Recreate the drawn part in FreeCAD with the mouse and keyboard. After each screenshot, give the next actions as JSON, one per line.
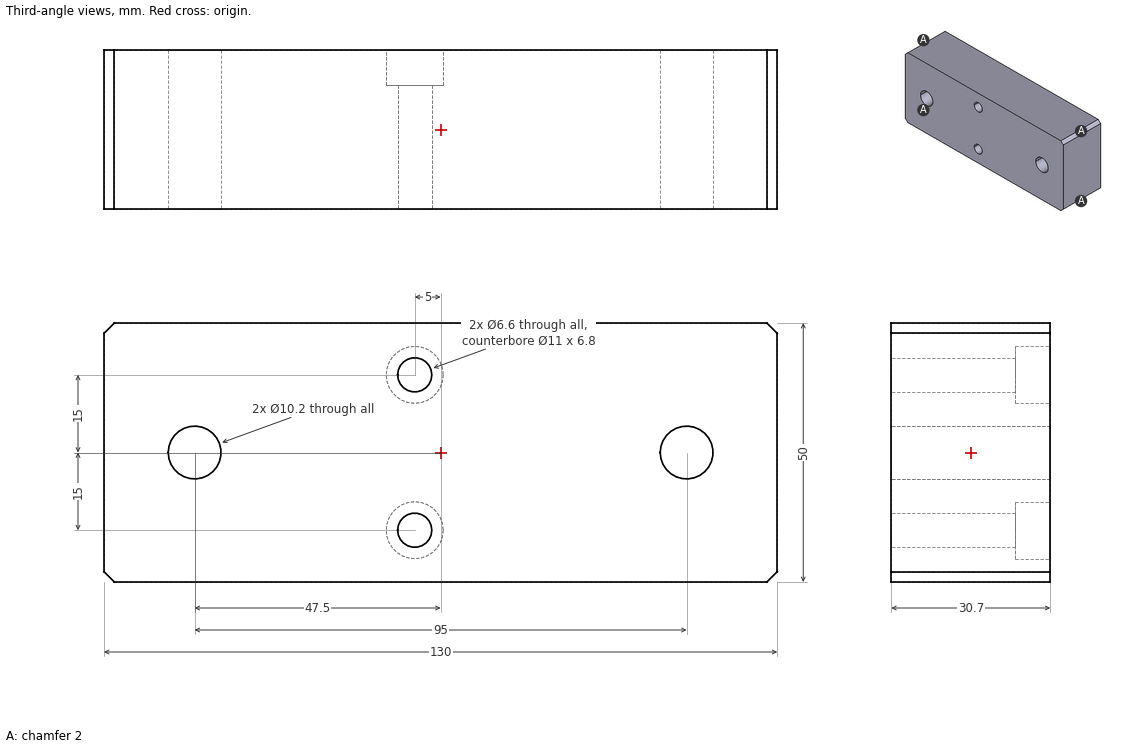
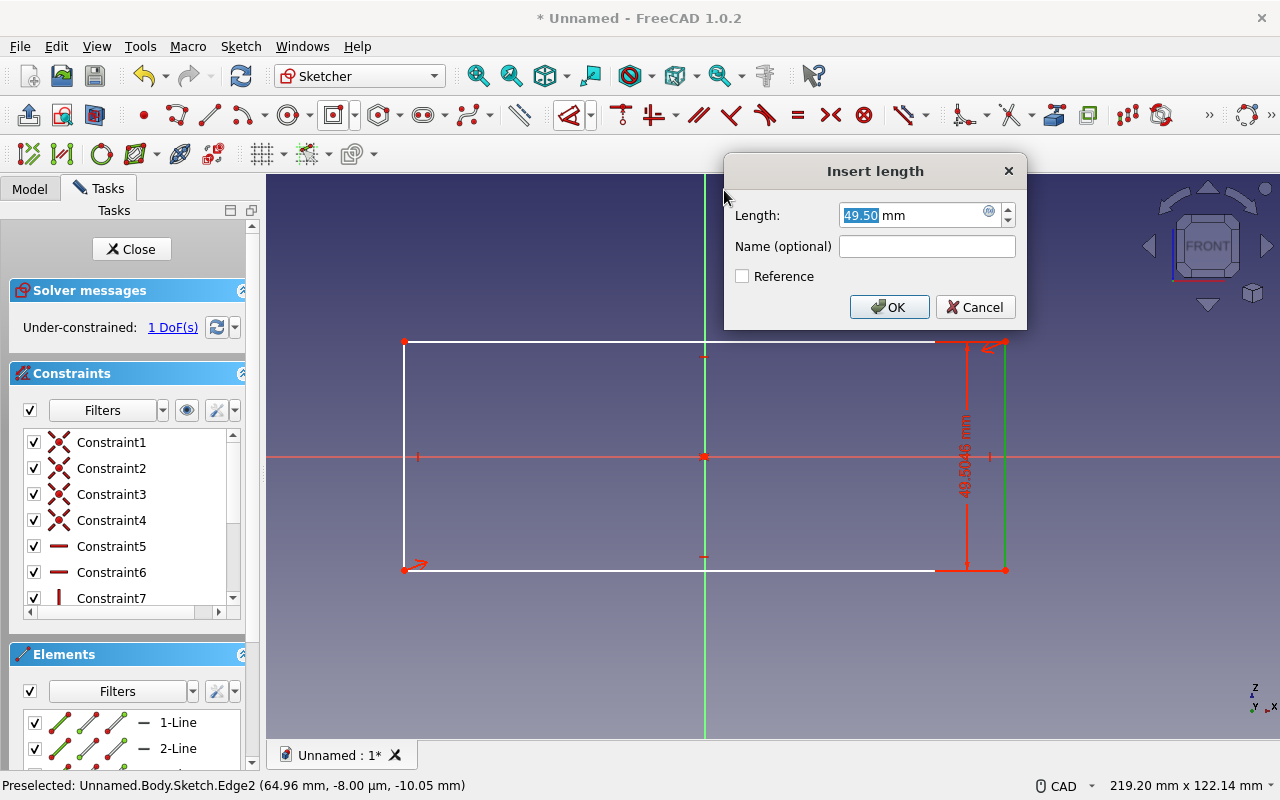
{"action": "type", "text": "50"}
{"action": "key", "text": "Return"}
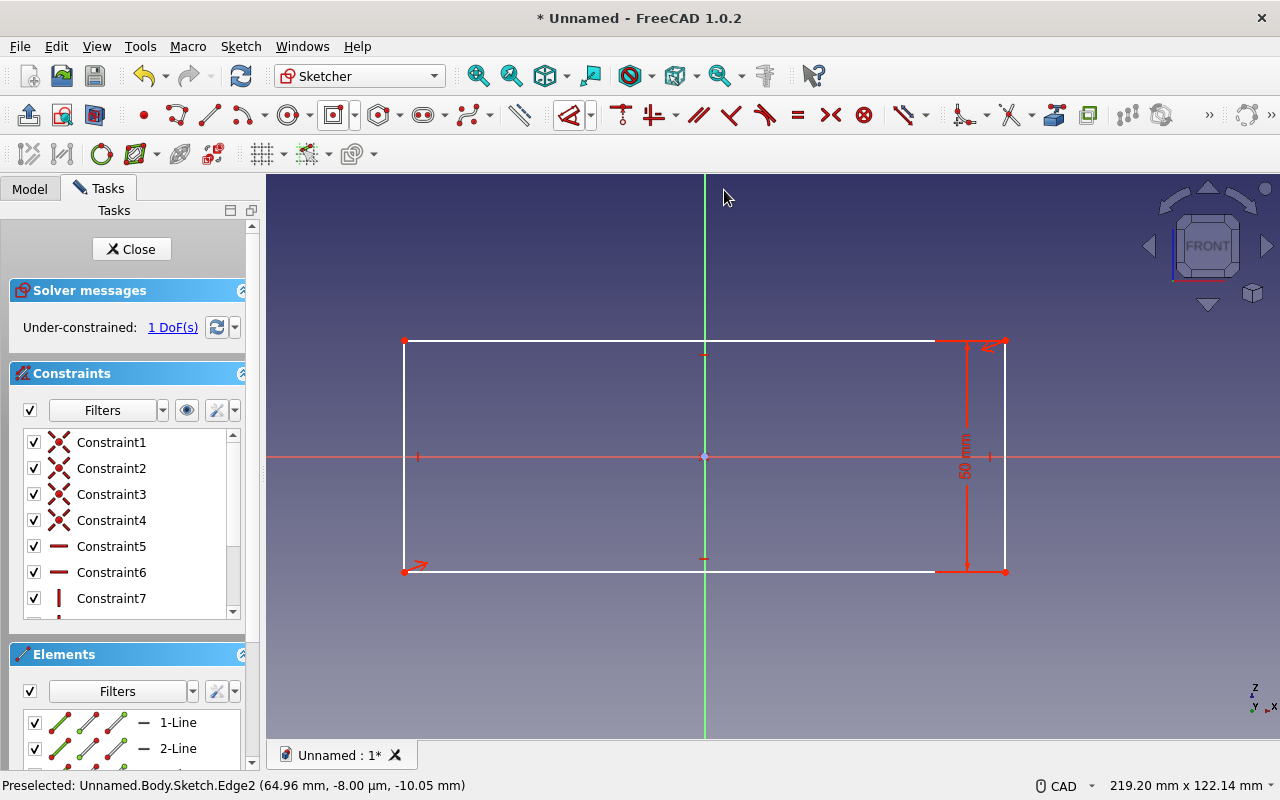
{"action": "left_click", "coordinate": [584, 572]}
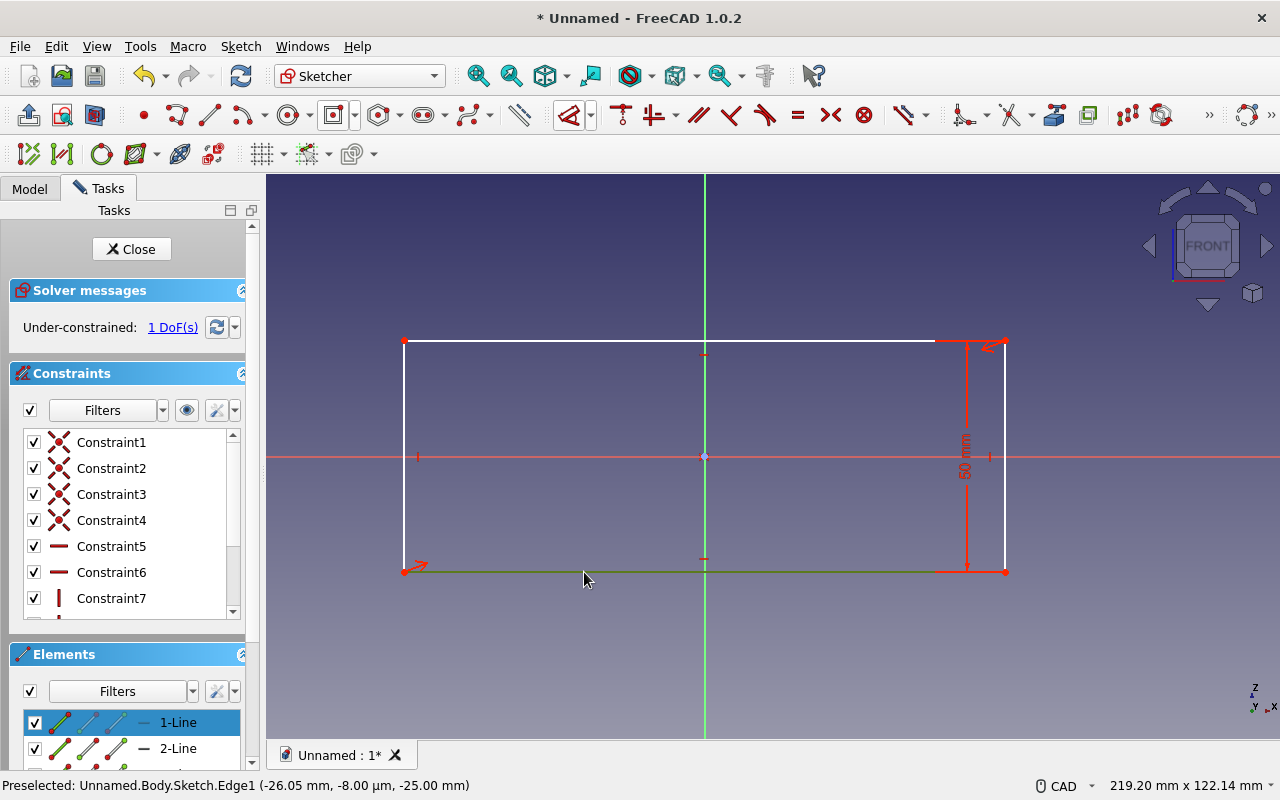
{"action": "key", "text": "l"}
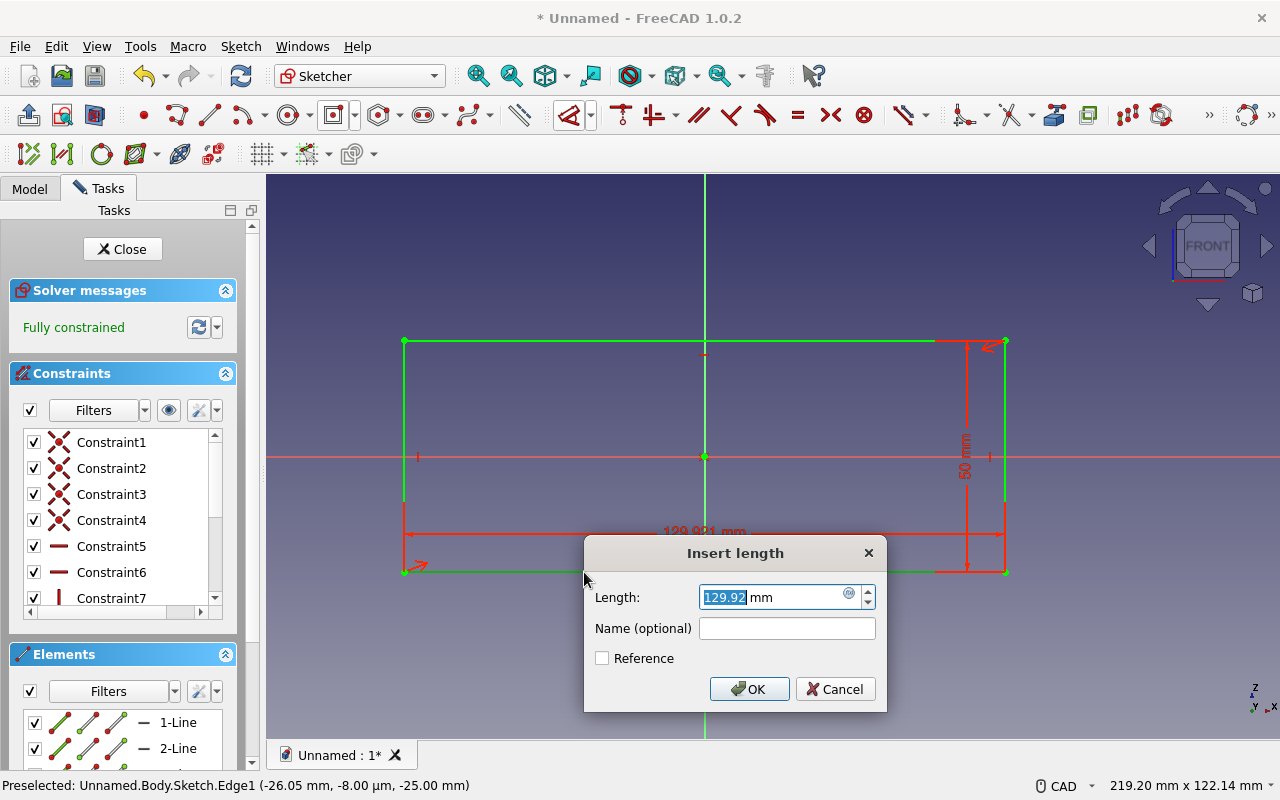
{"action": "type", "text": "130"}
{"action": "key", "text": "Return"}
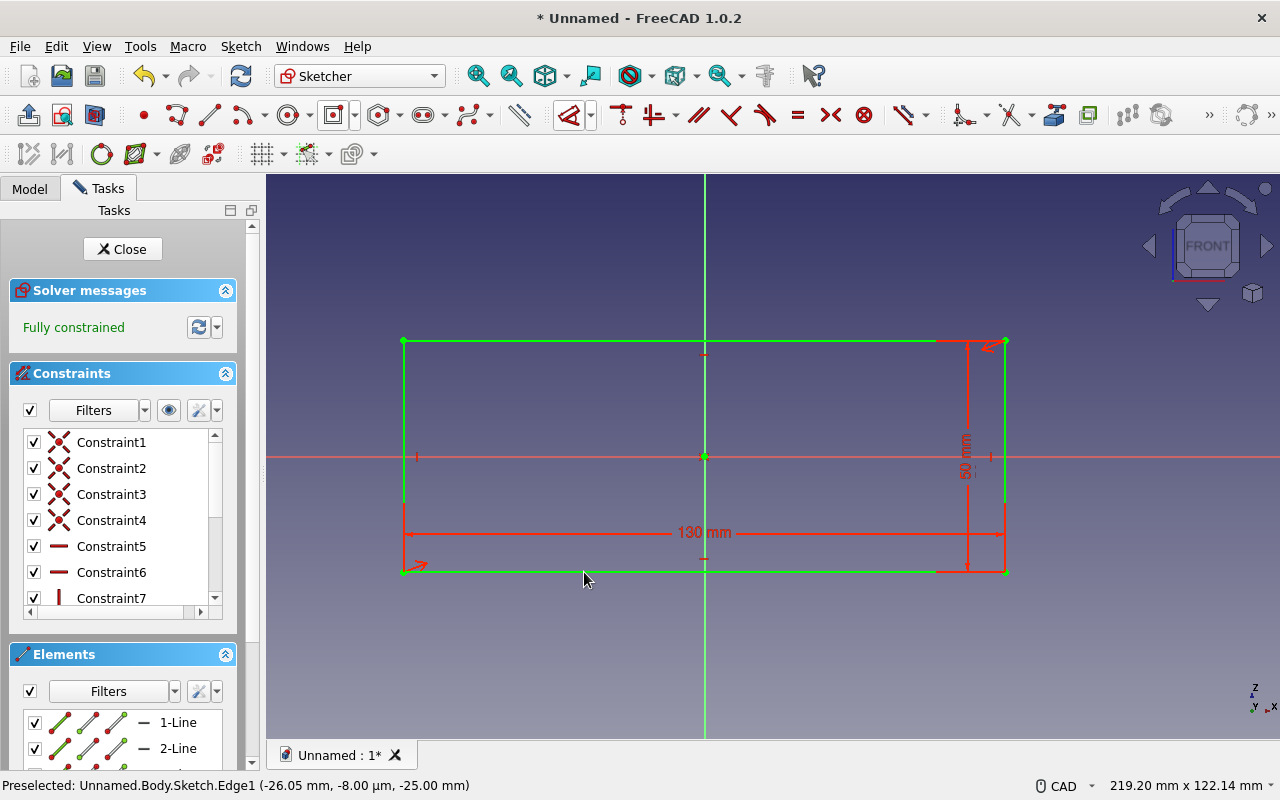
{"action": "left_click", "coordinate": [123, 249]}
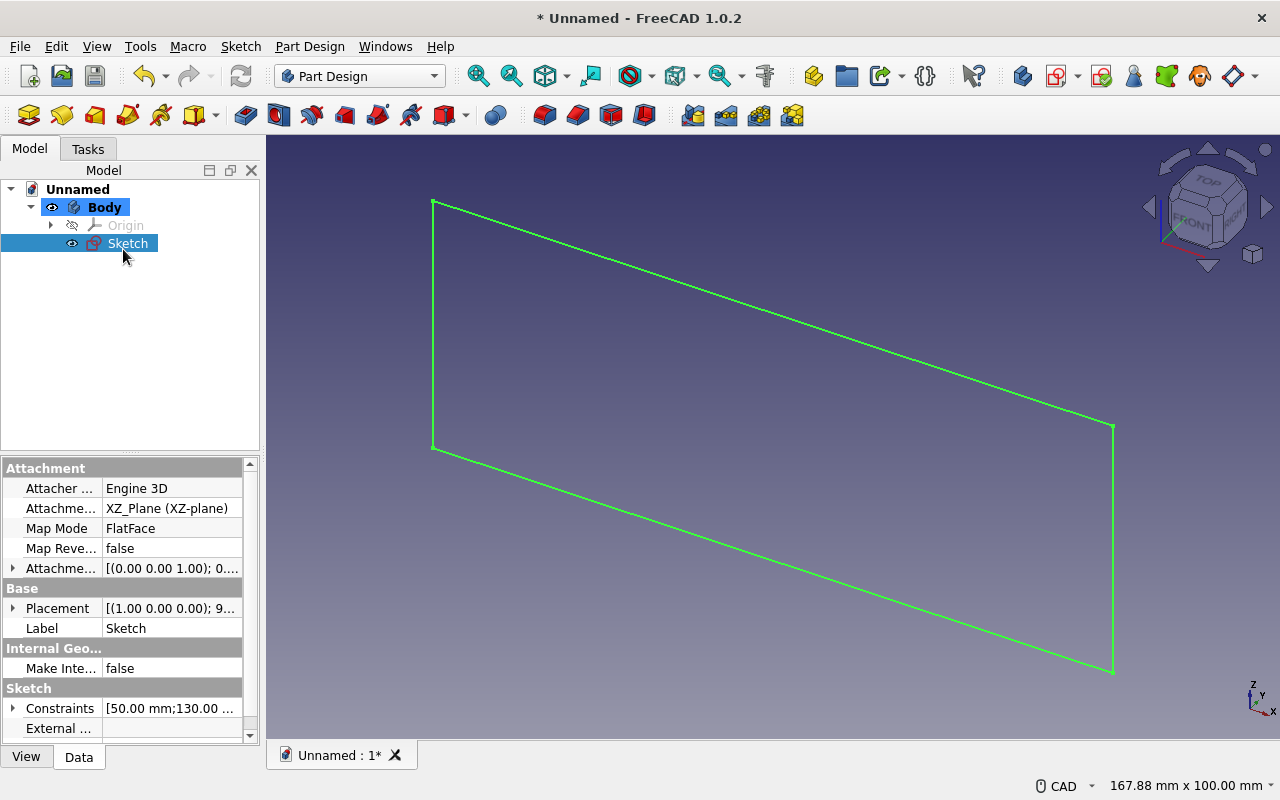
{"action": "left_click", "coordinate": [29, 116]}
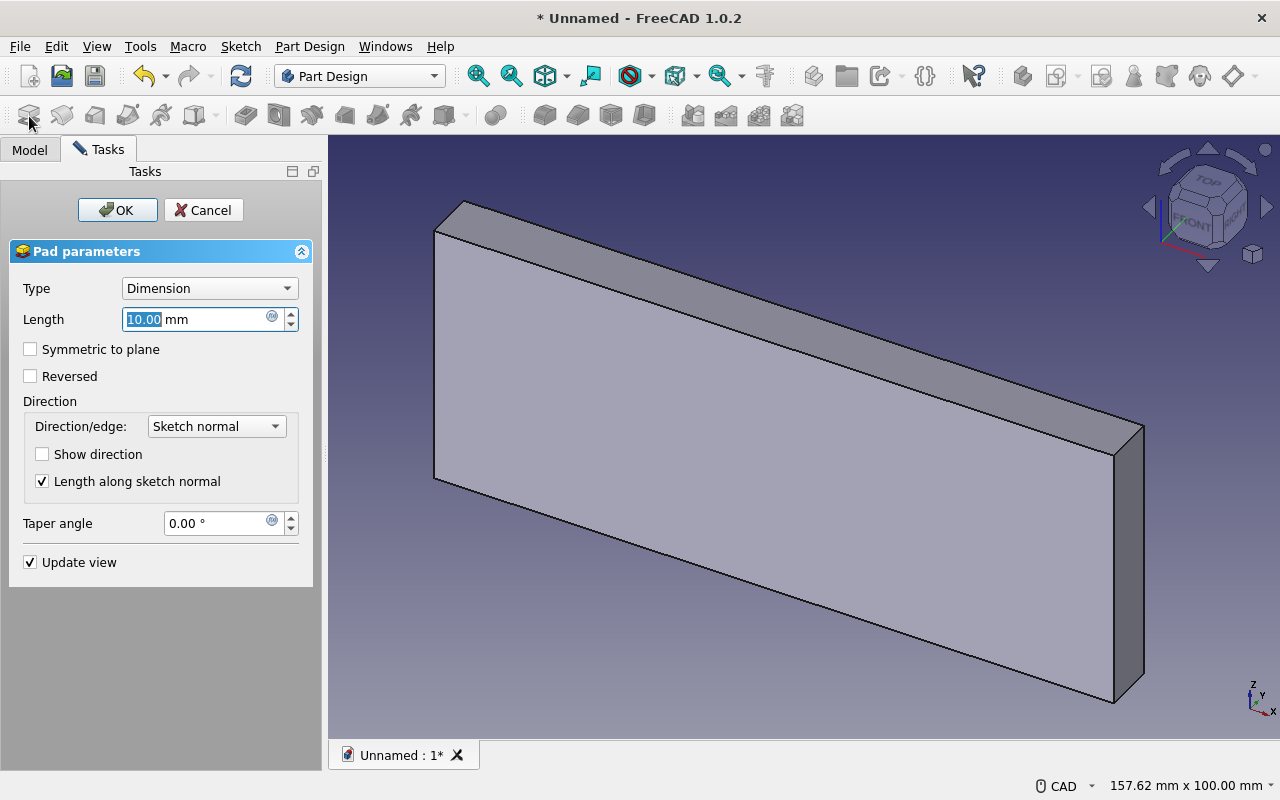
{"action": "type", "text": "30.7"}
{"action": "key", "text": "Tab"}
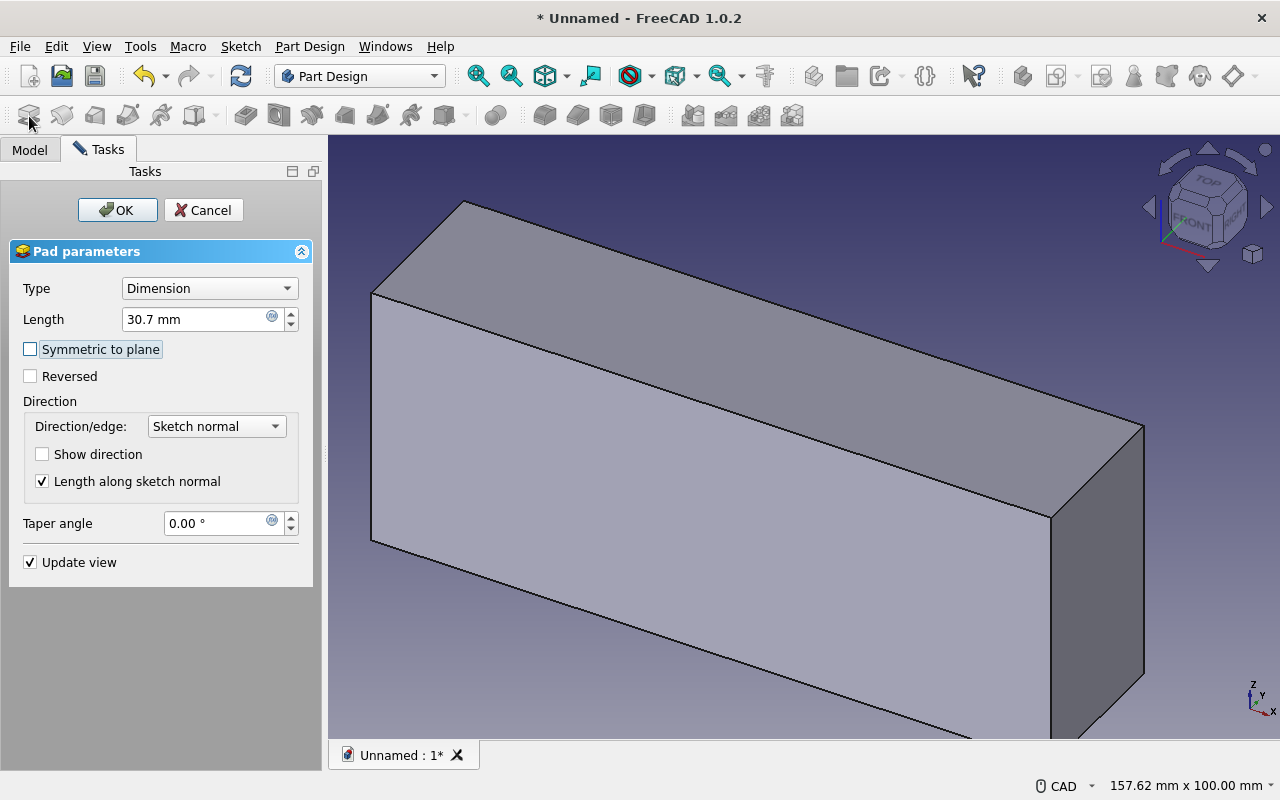
{"action": "left_click", "coordinate": [31, 349]}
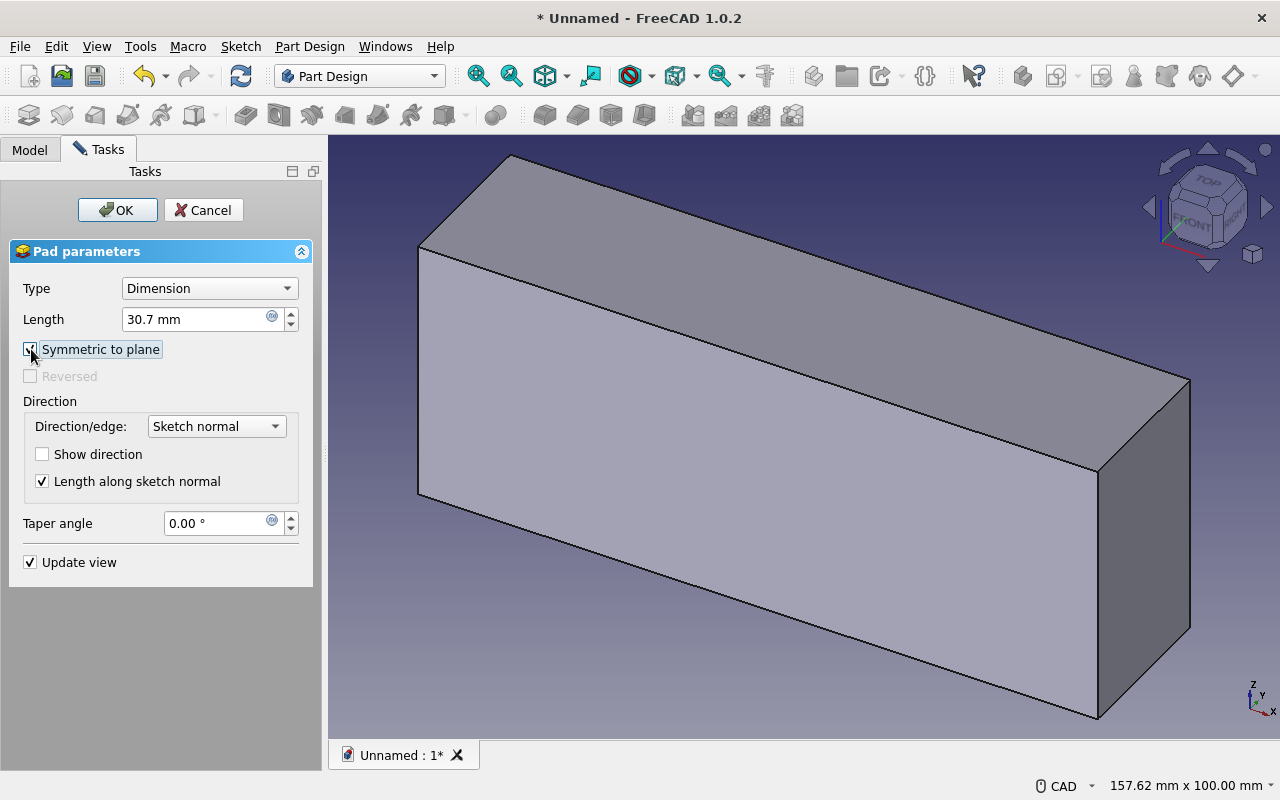
{"action": "left_click", "coordinate": [118, 210]}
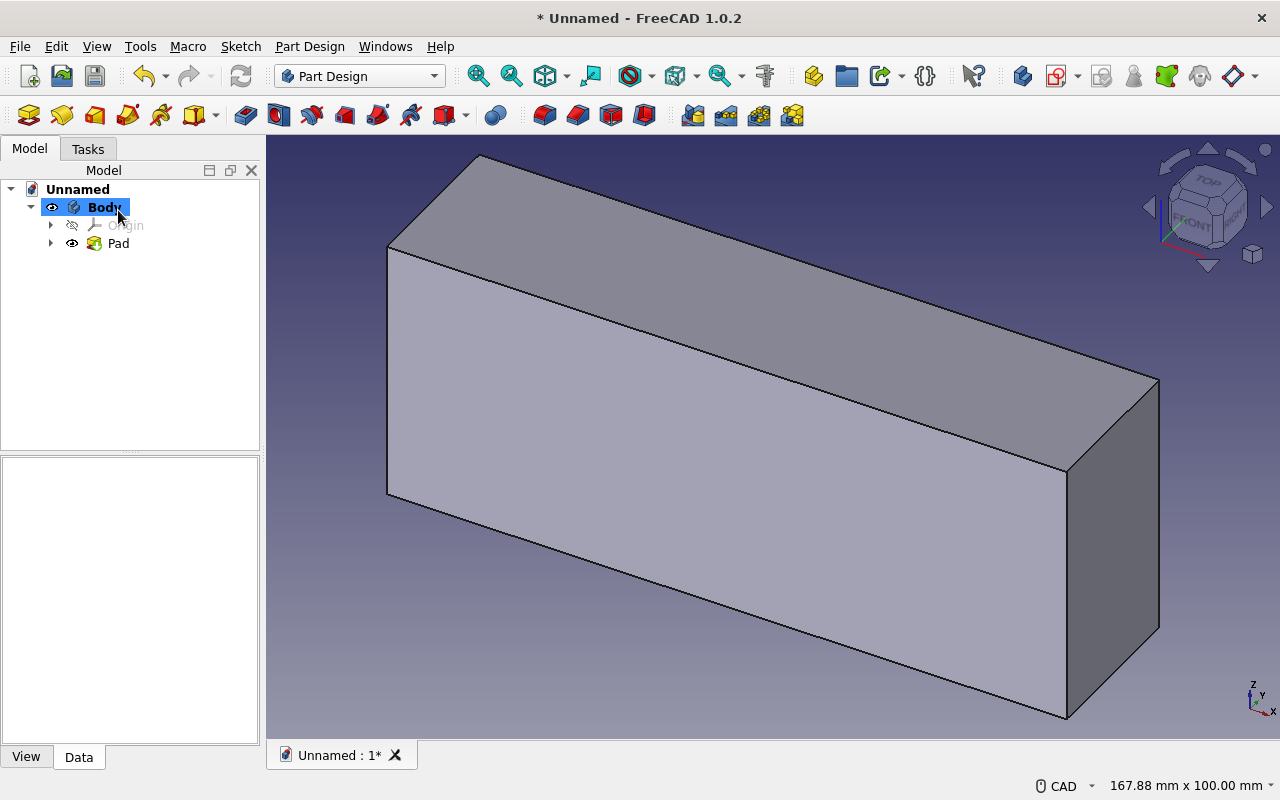
{"action": "left_click", "coordinate": [1113, 425]}